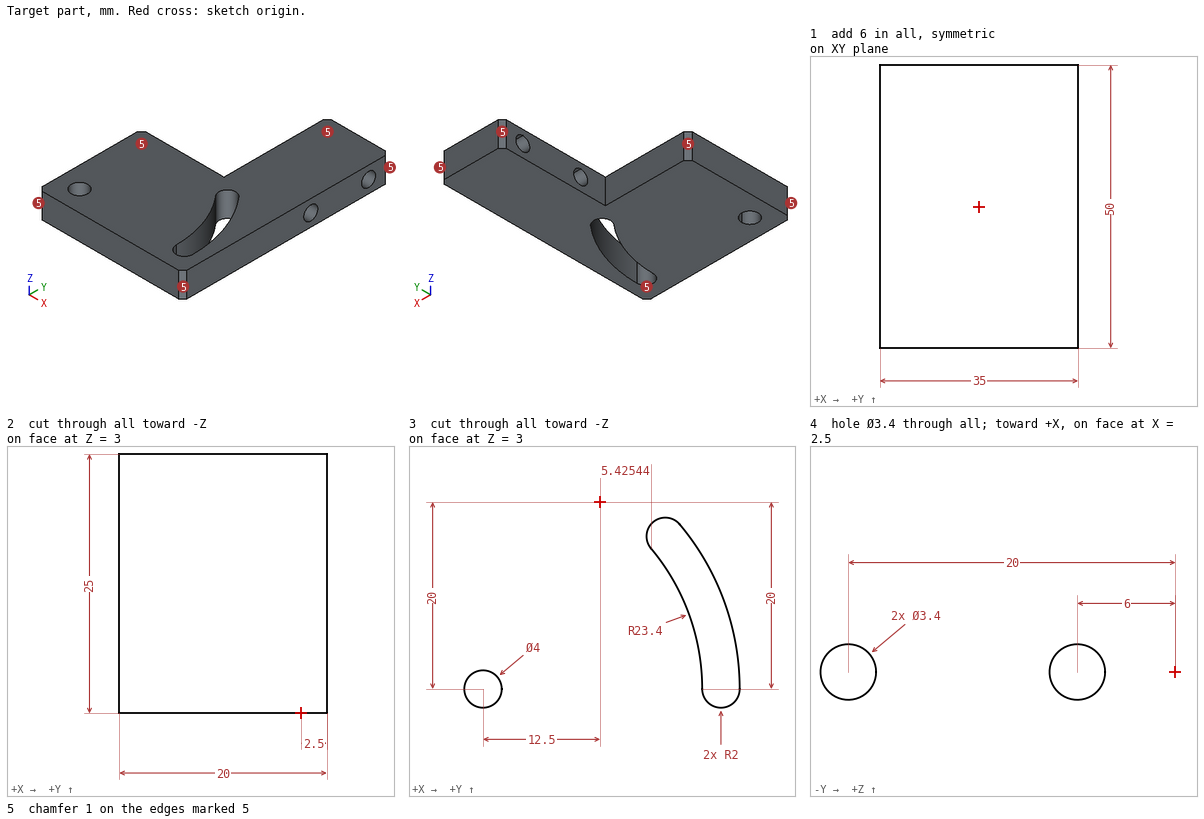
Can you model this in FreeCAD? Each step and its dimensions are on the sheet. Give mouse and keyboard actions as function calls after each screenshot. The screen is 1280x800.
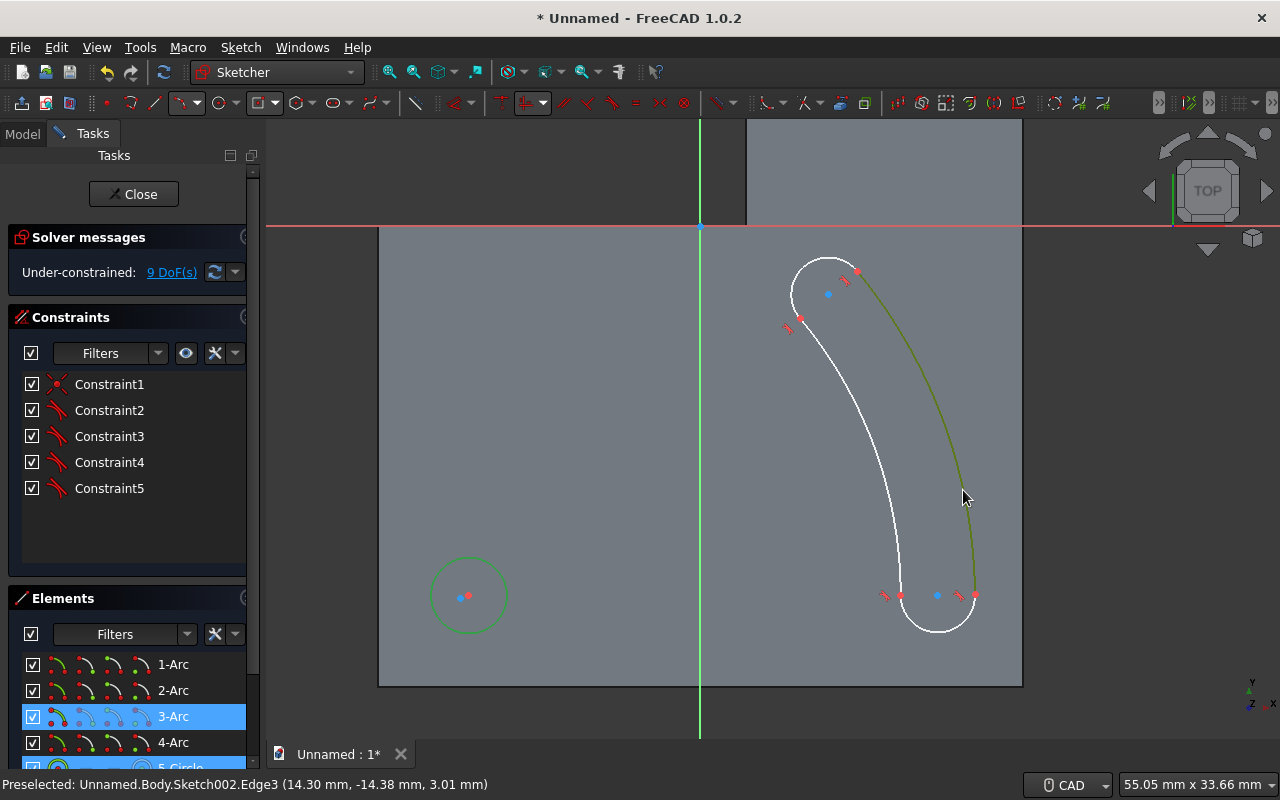
click(502, 104)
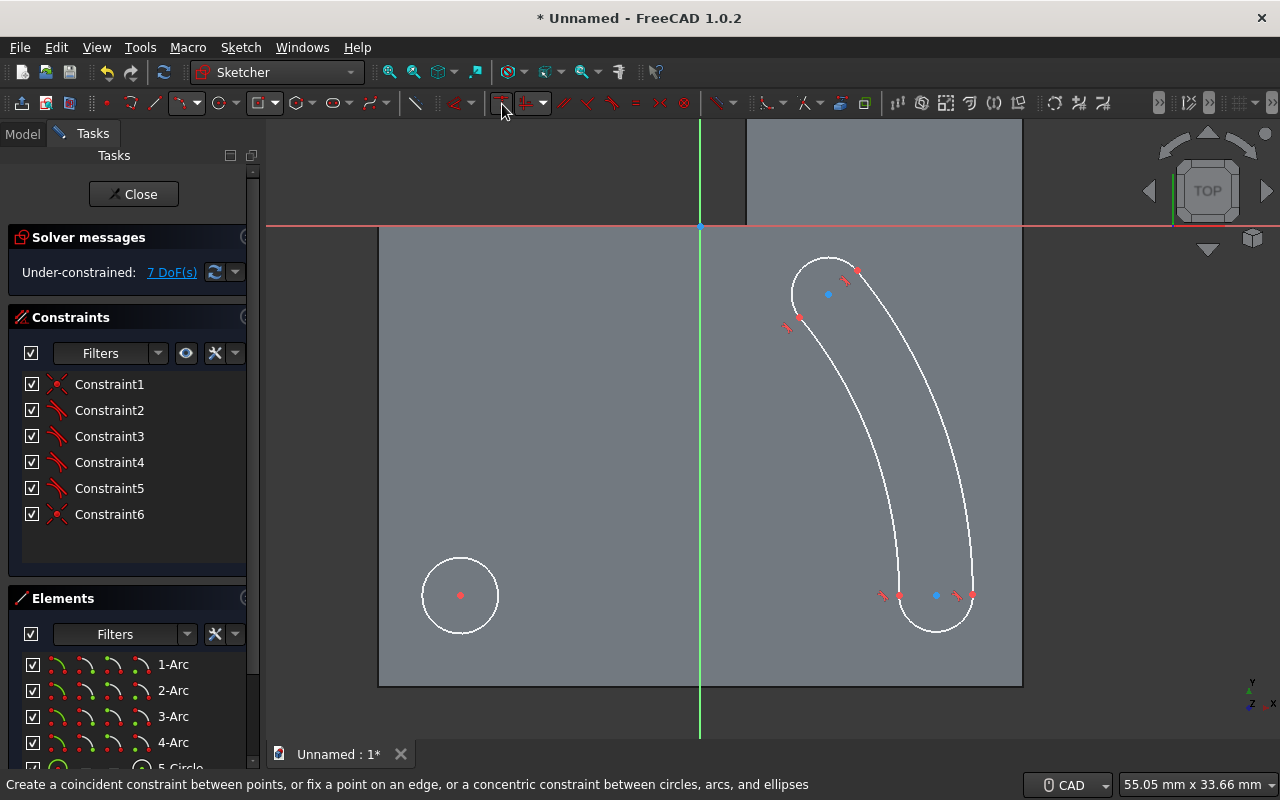
click(454, 104)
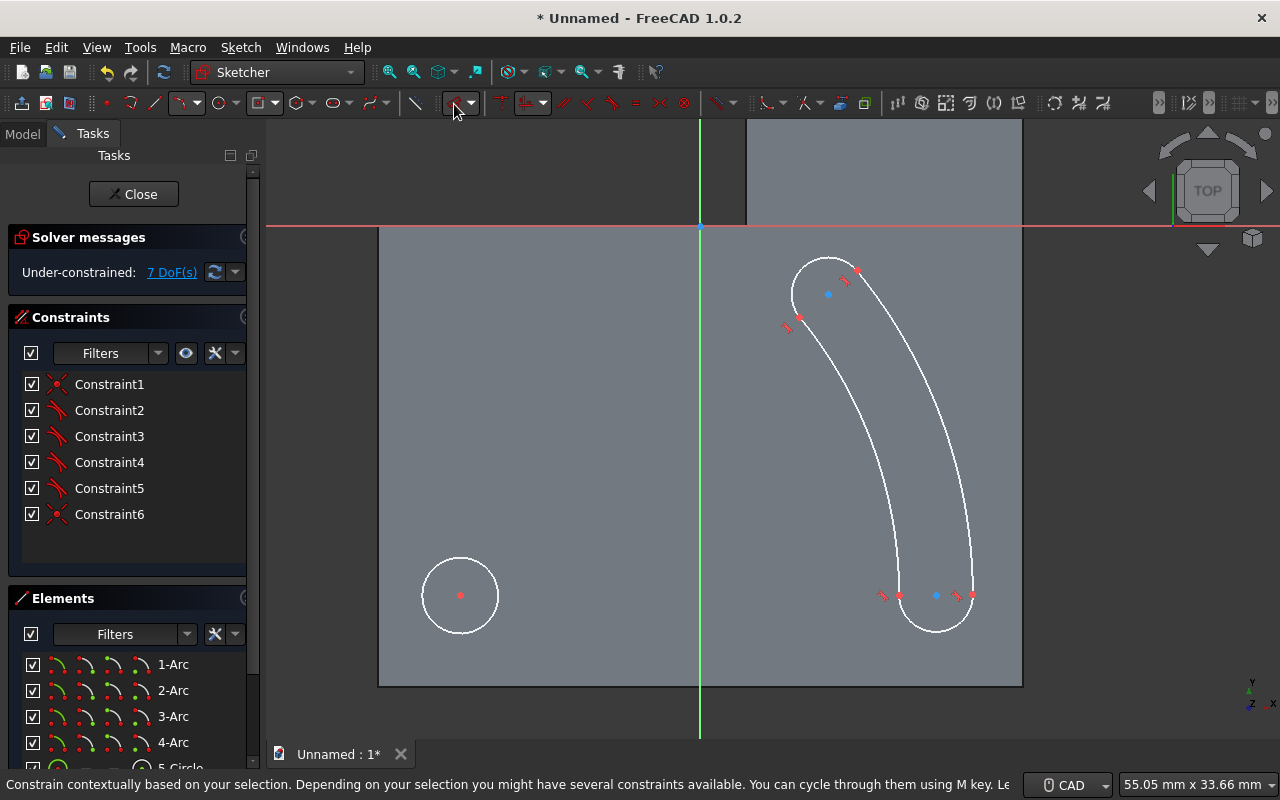
click(890, 506)
click(921, 499)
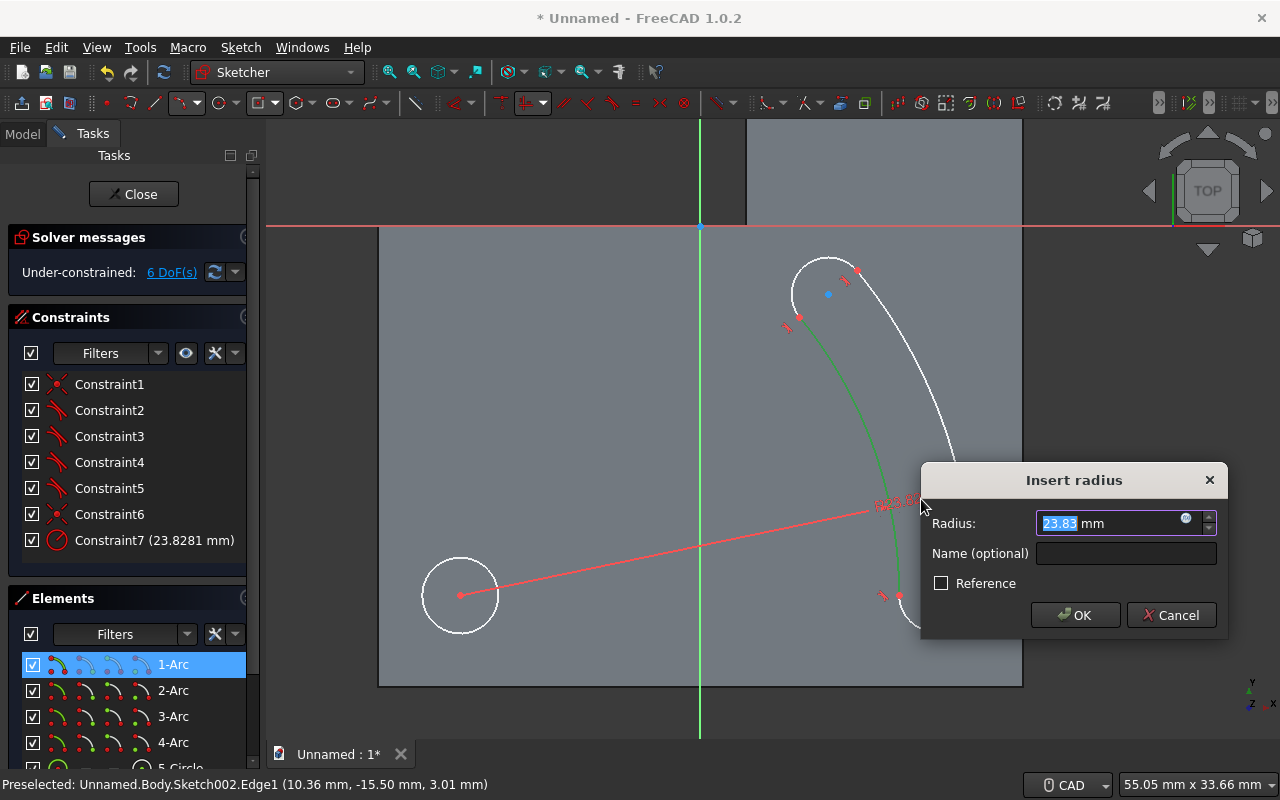
text(23.4)
key(Return)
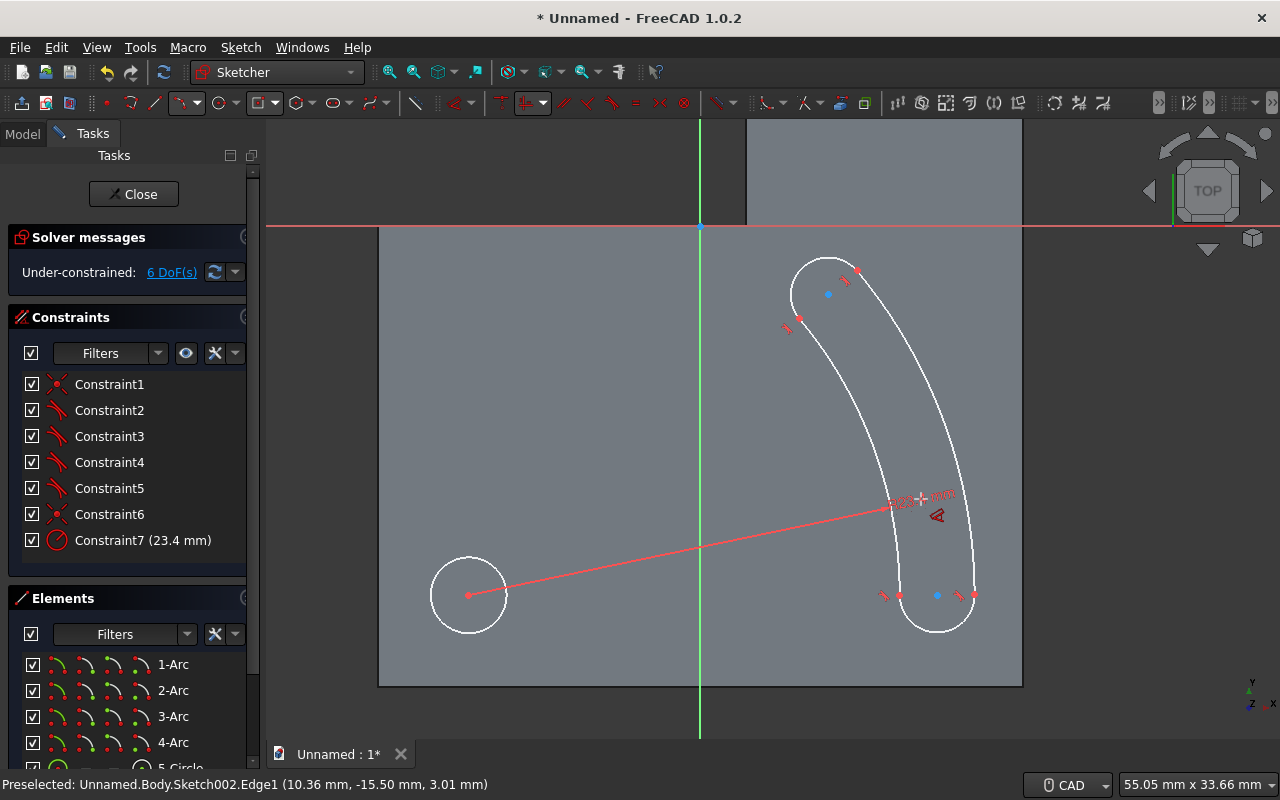
click(915, 625)
click(896, 651)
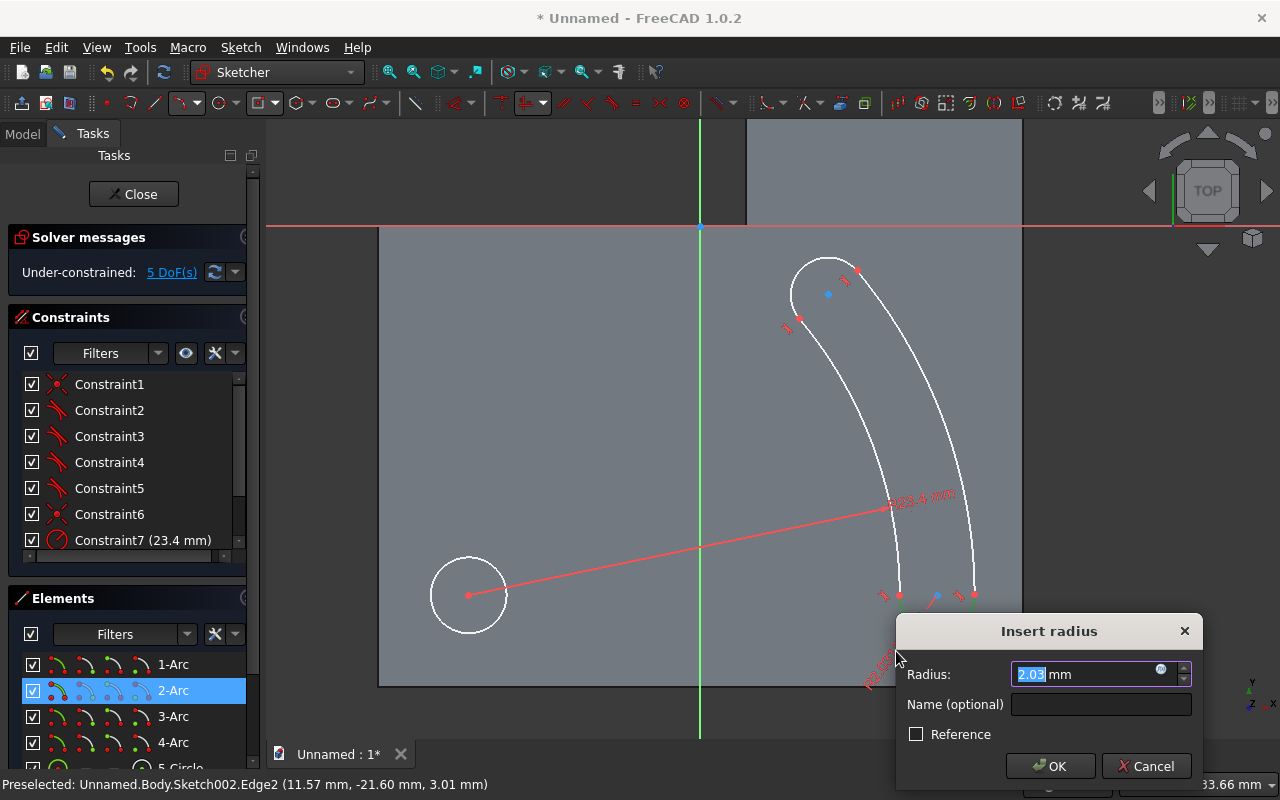
text(2)
key(Return)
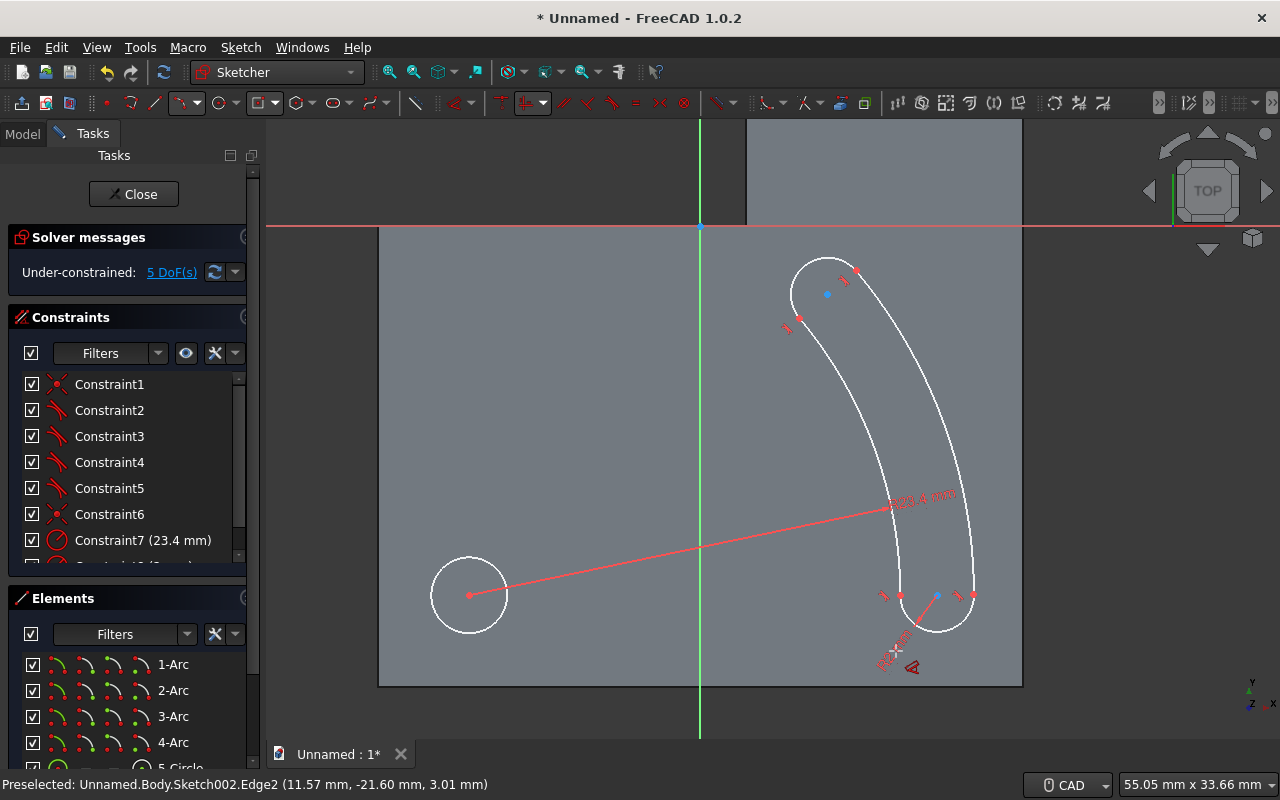
click(496, 568)
click(518, 545)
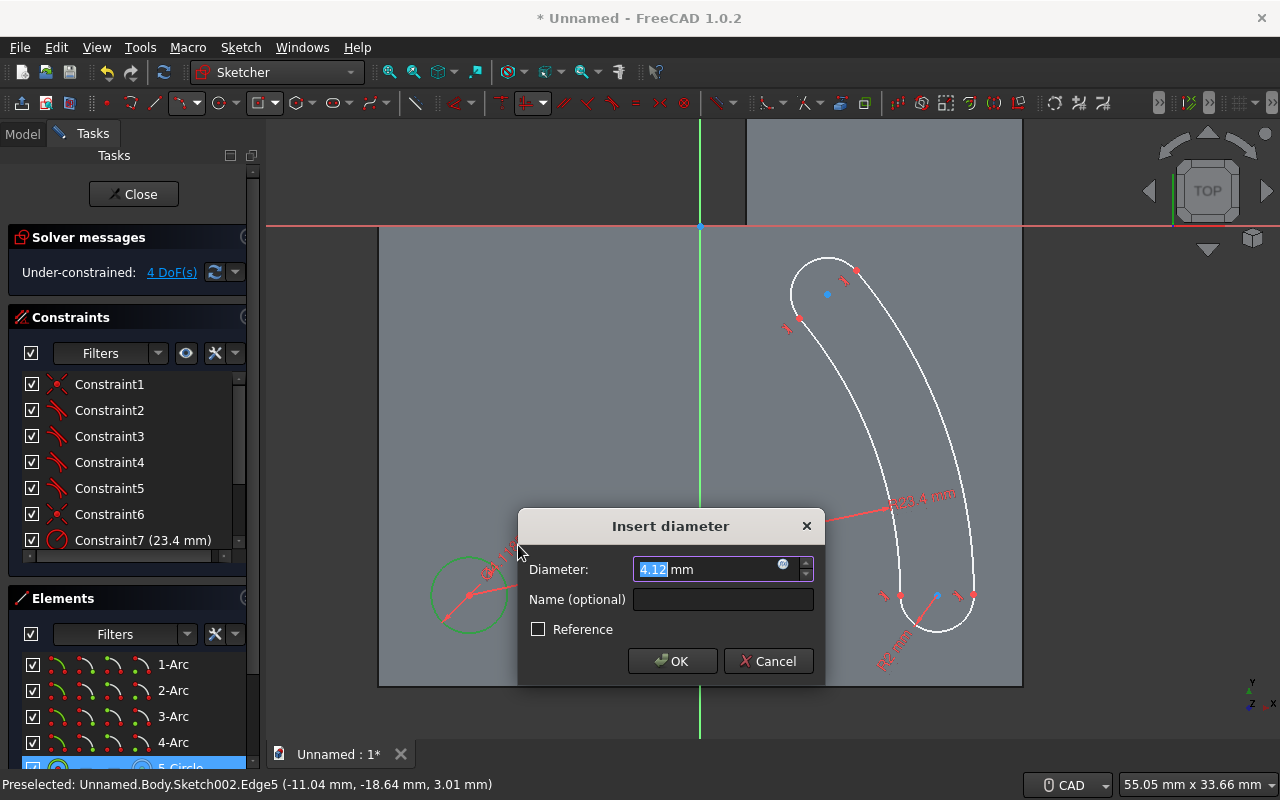
text(4)
key(Return)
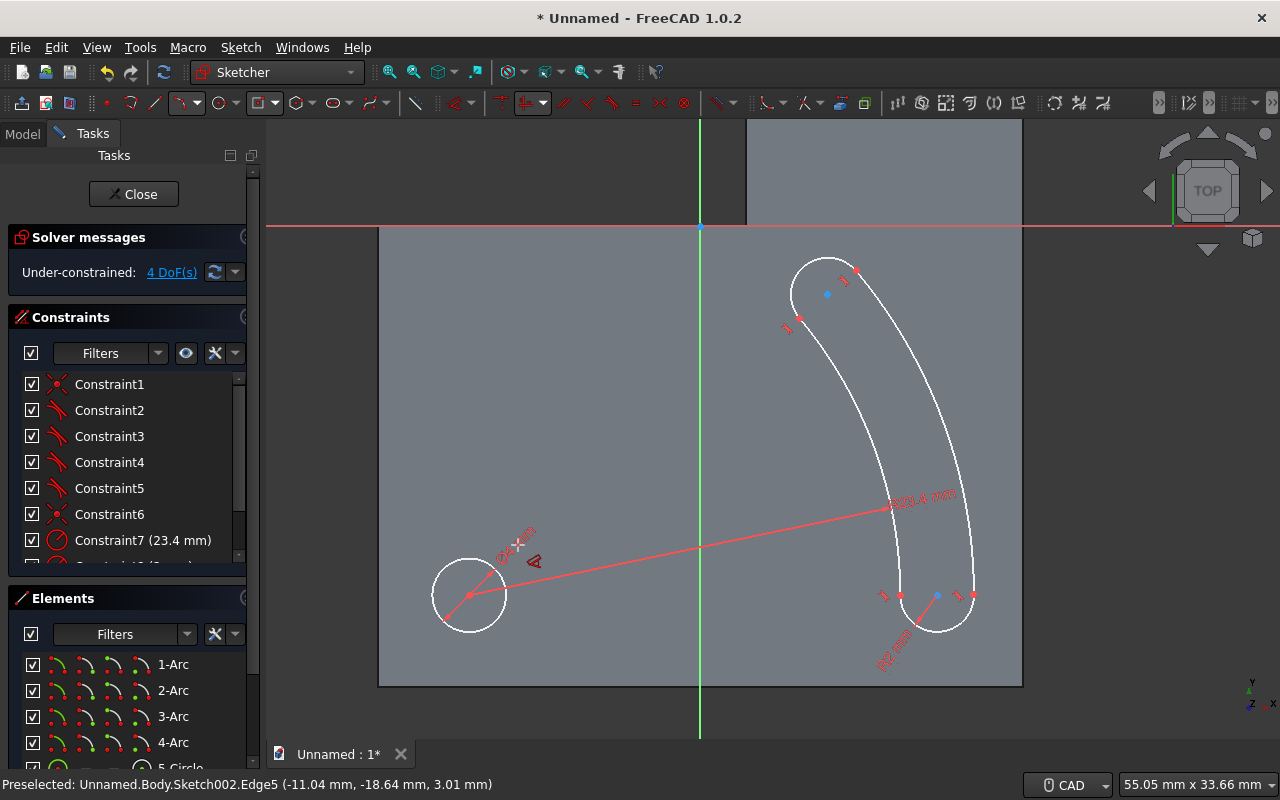
click(469, 595)
click(435, 411)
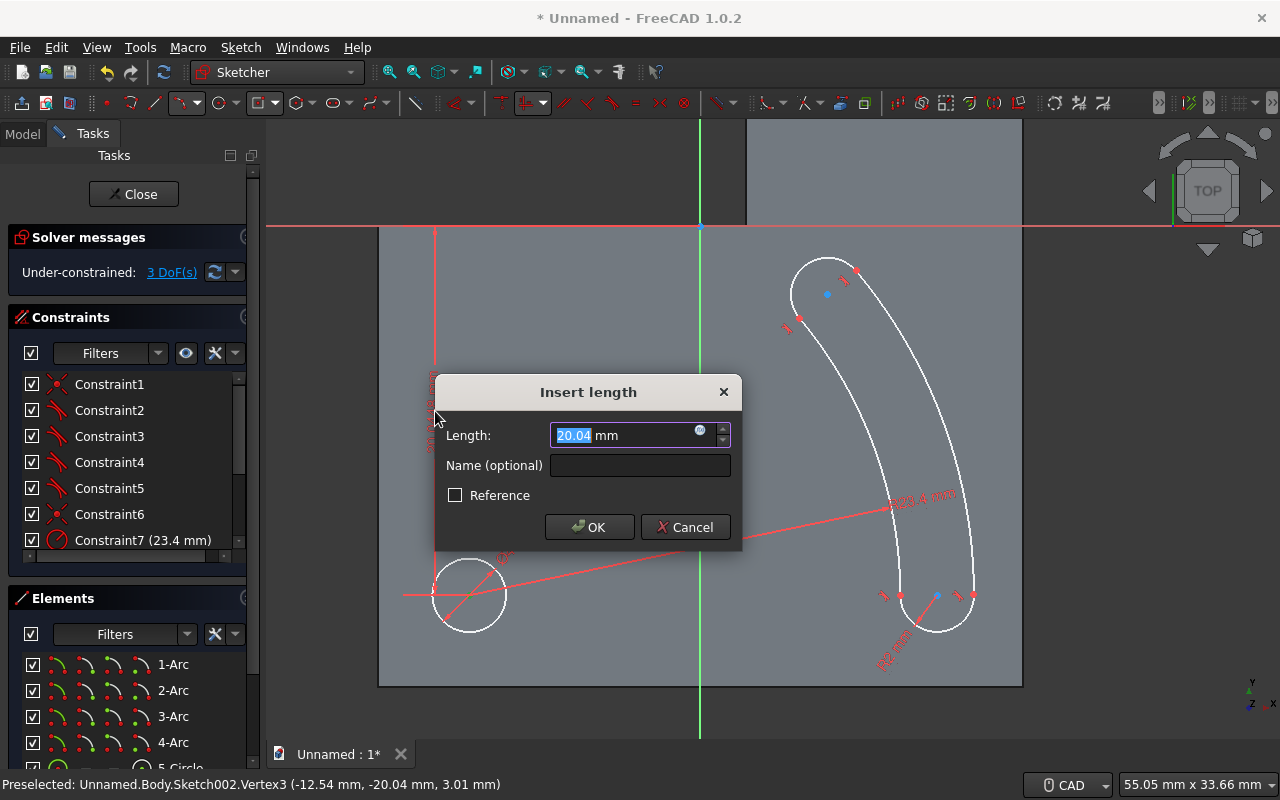
text(20)
key(Return)